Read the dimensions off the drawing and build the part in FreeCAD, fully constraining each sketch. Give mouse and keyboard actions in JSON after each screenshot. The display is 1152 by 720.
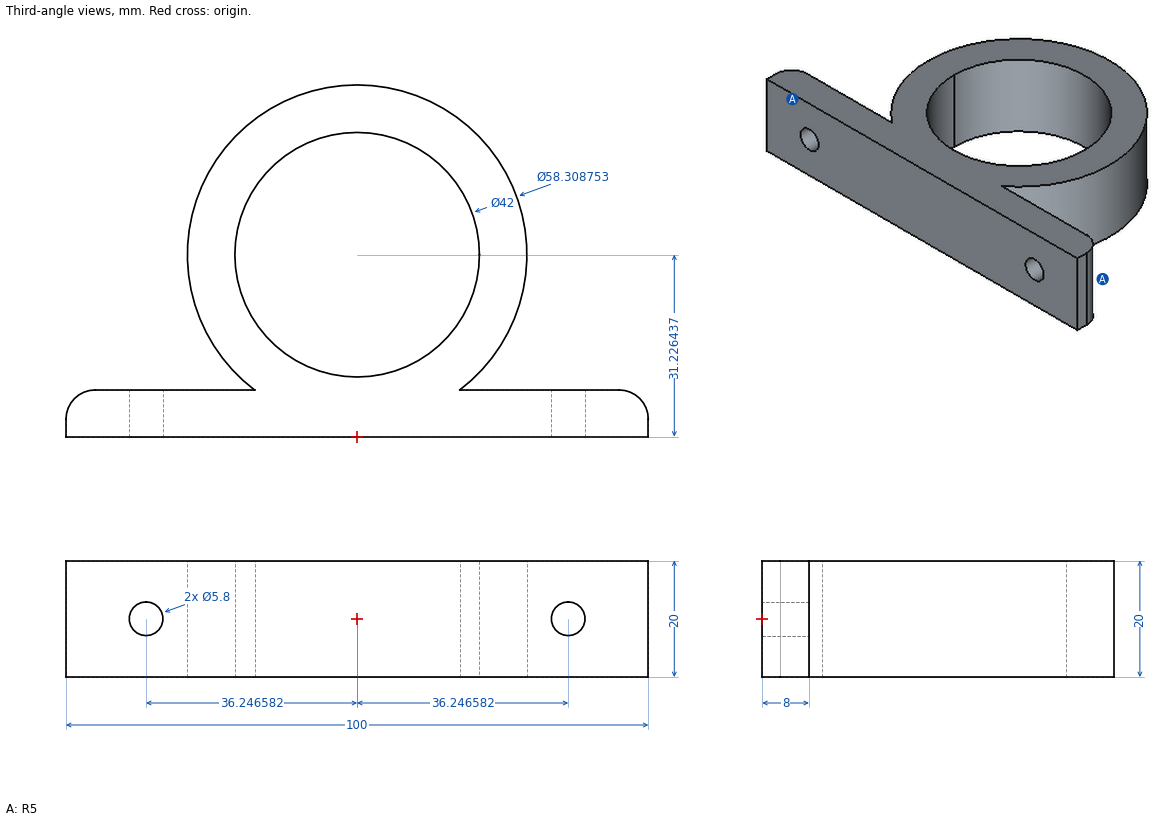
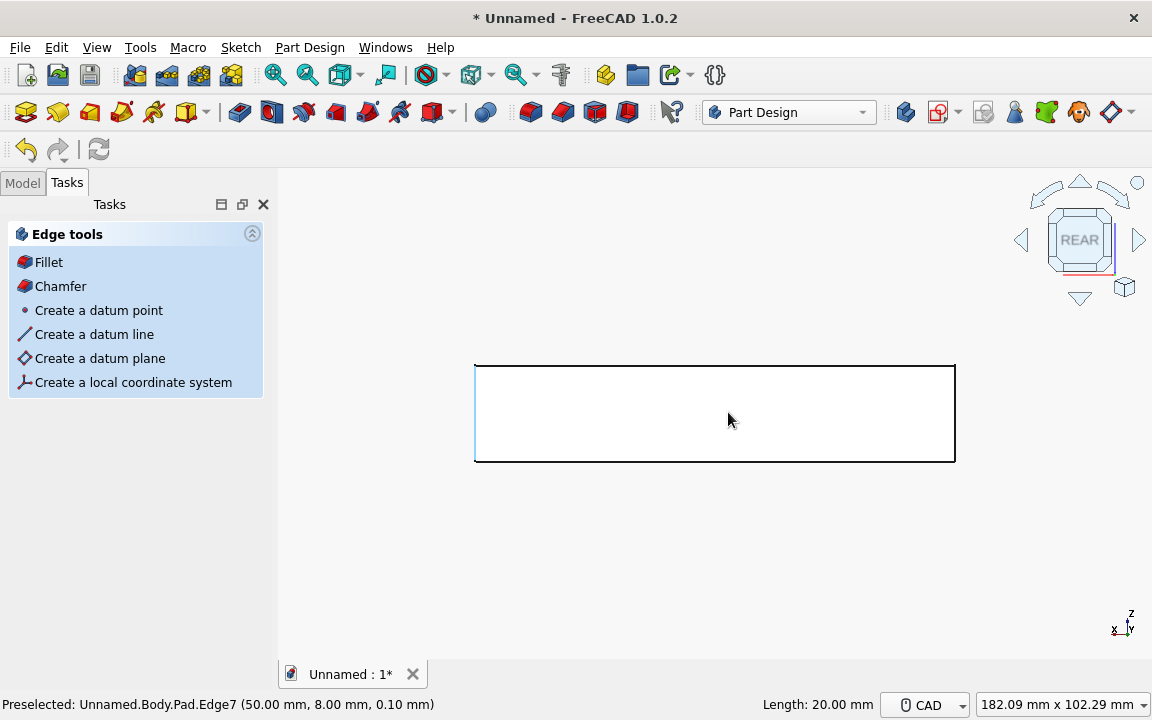
{"action": "left_click", "coordinate": [955, 412], "text": "ctrl"}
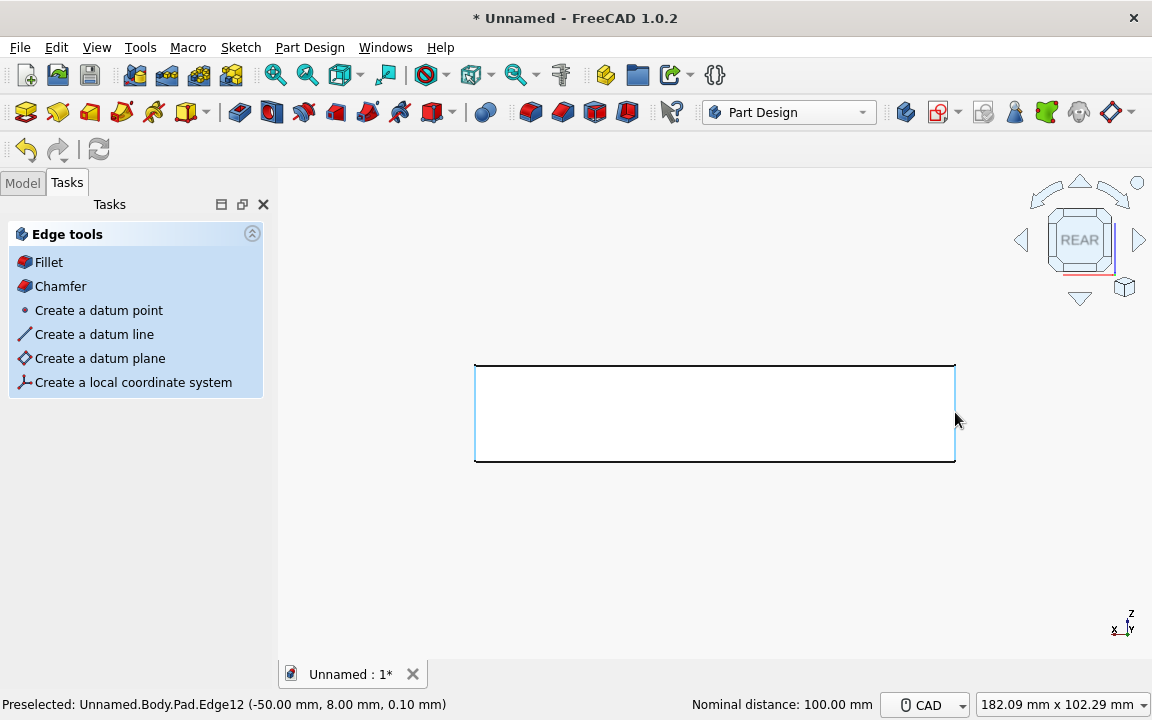
{"action": "left_click", "coordinate": [532, 112]}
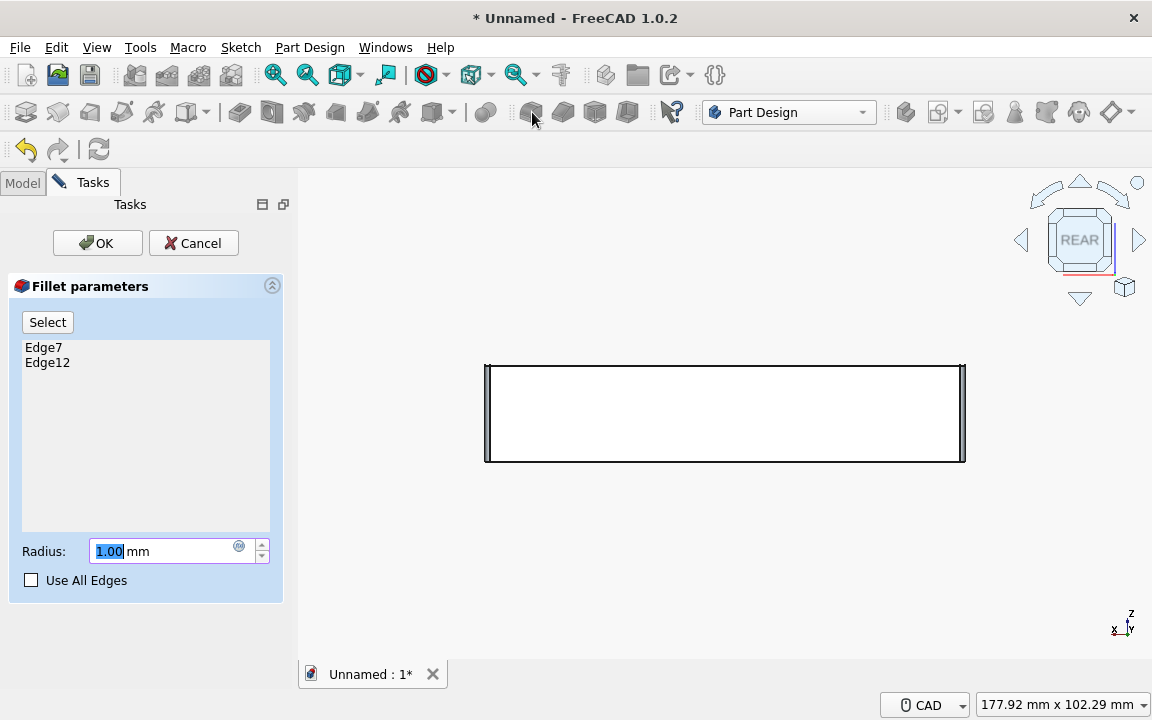
{"action": "type", "text": "5"}
{"action": "key", "text": "Tab"}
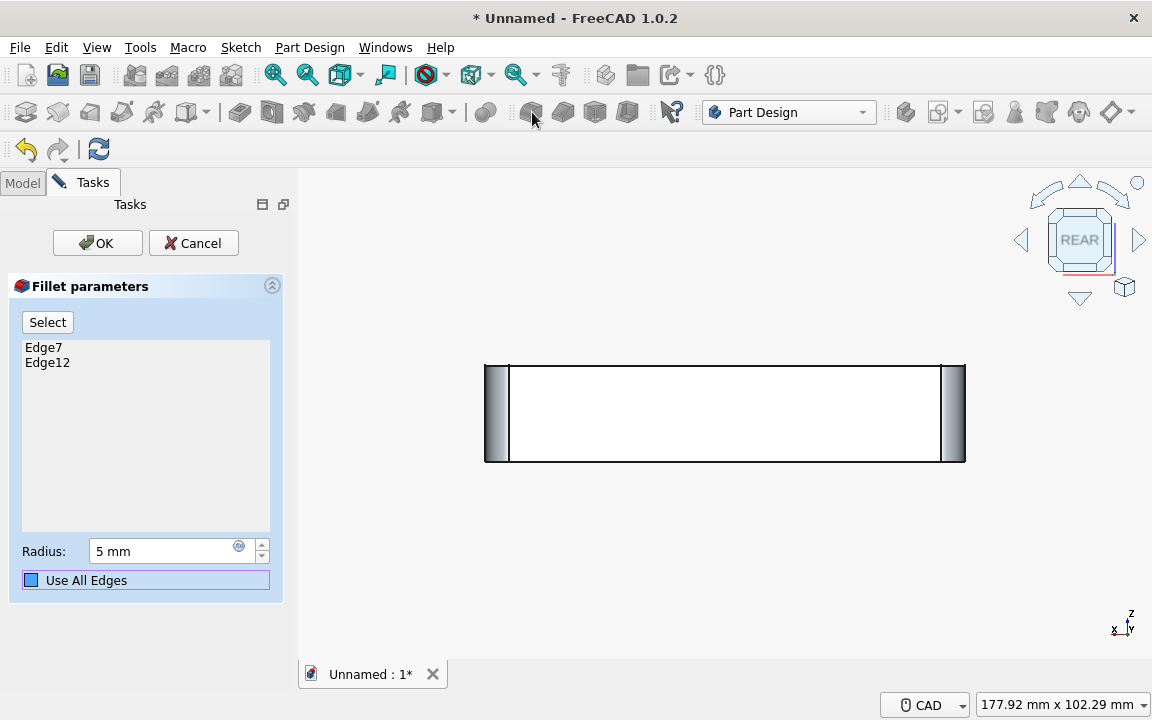
{"action": "left_click", "coordinate": [98, 243]}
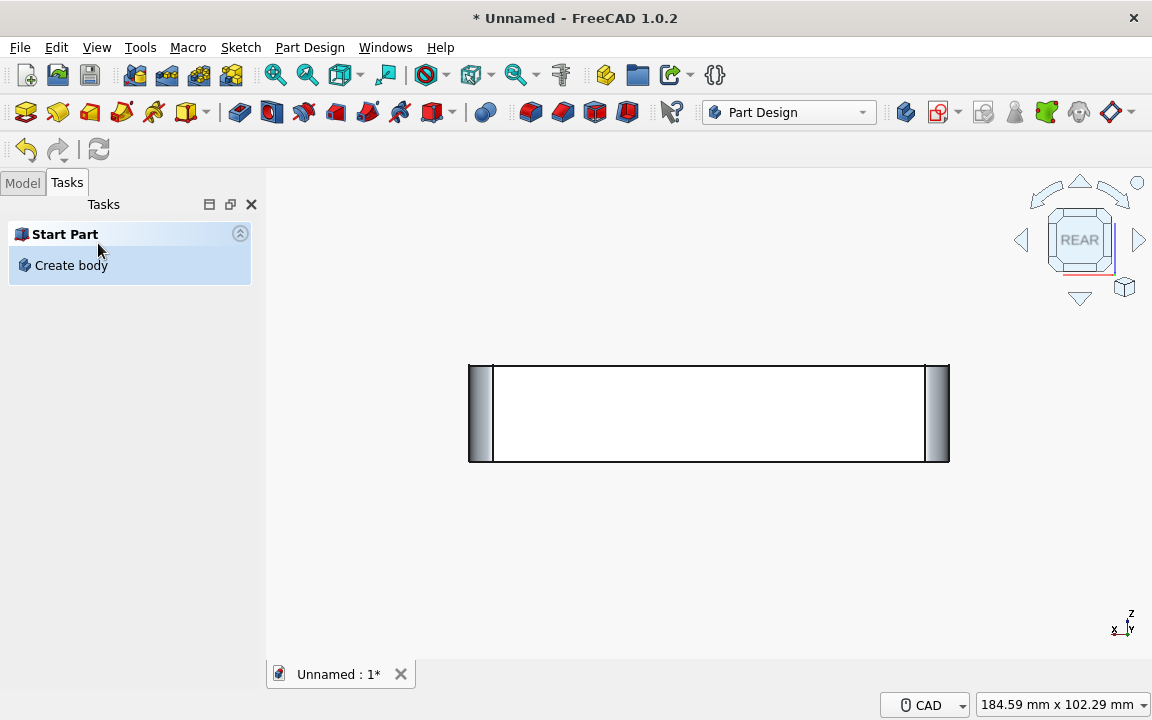
{"action": "key", "text": "0"}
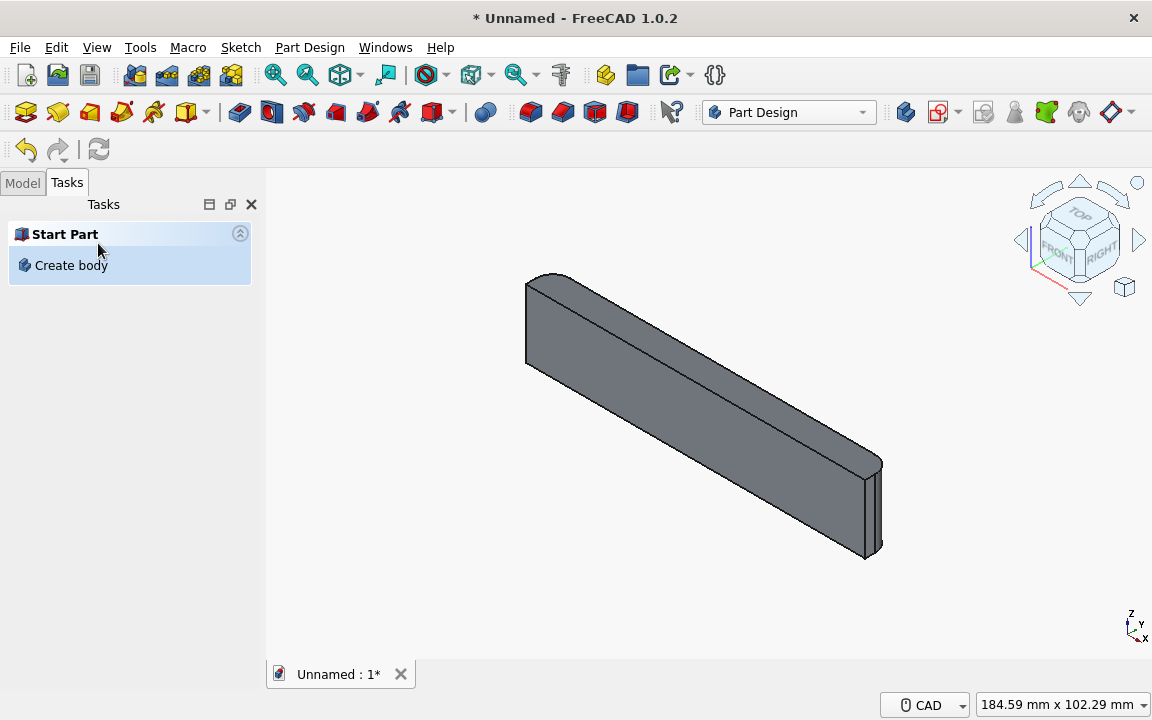
{"action": "left_click", "coordinate": [854, 457]}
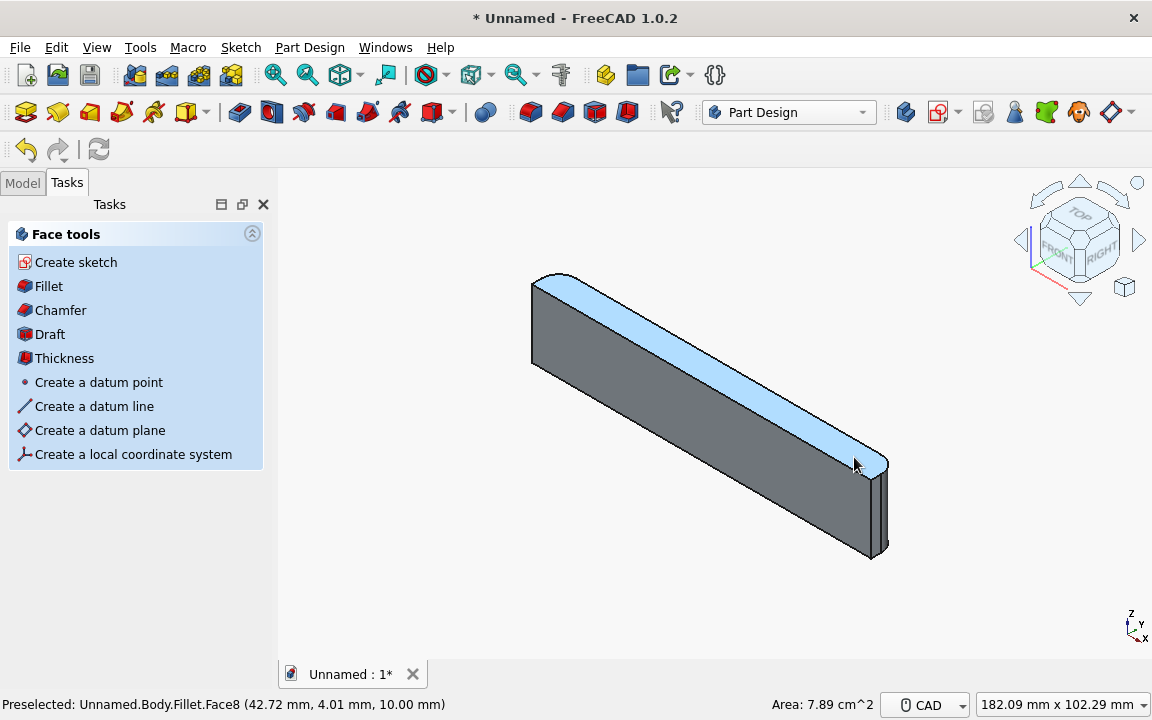
{"action": "left_click", "coordinate": [938, 112]}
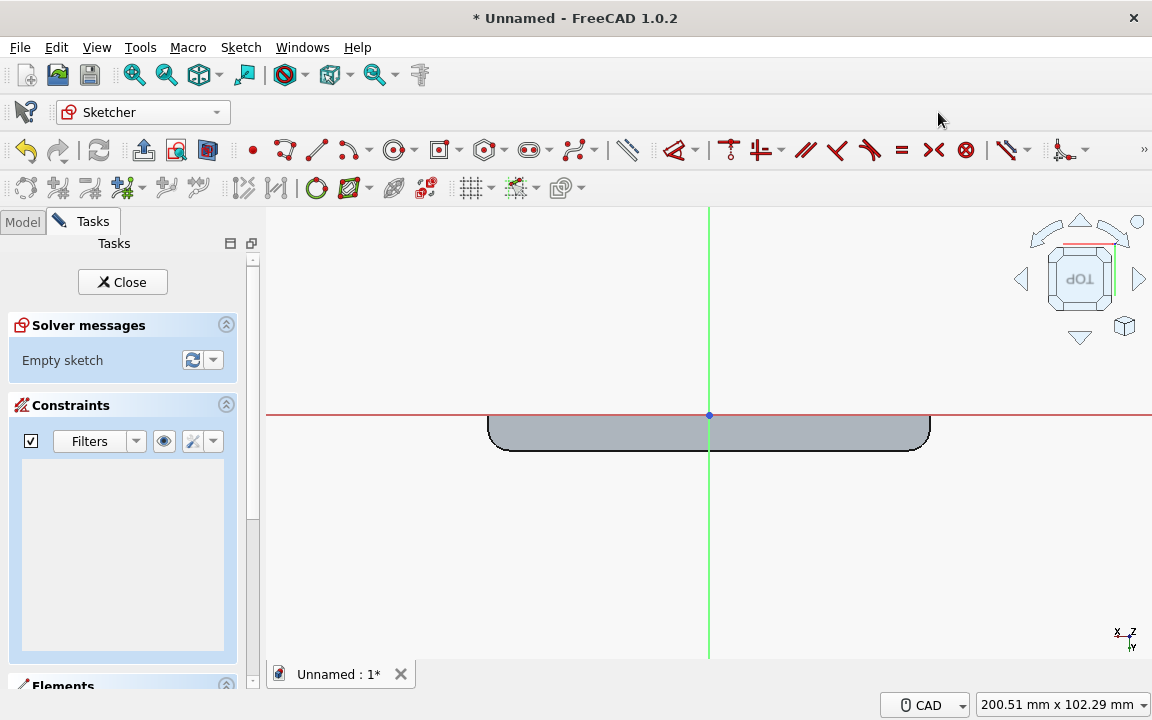
{"action": "scroll", "coordinate": [331, 235], "scroll_direction": "down", "scroll_amount": 1}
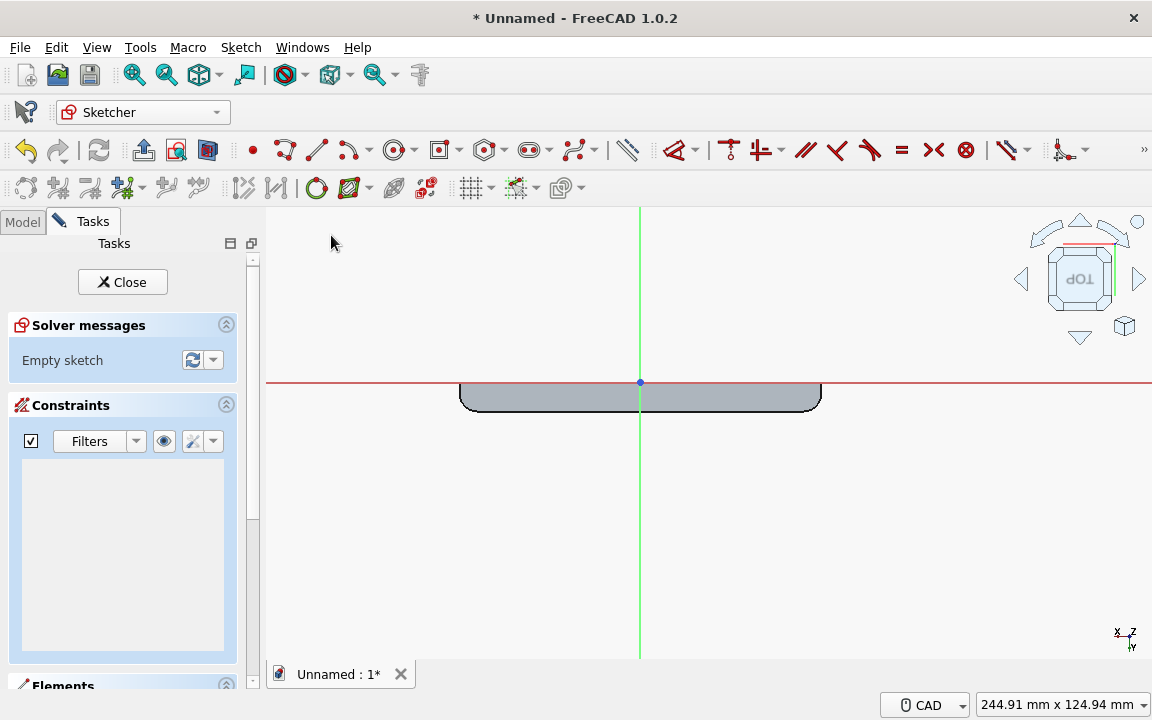
{"action": "left_click", "coordinate": [394, 150]}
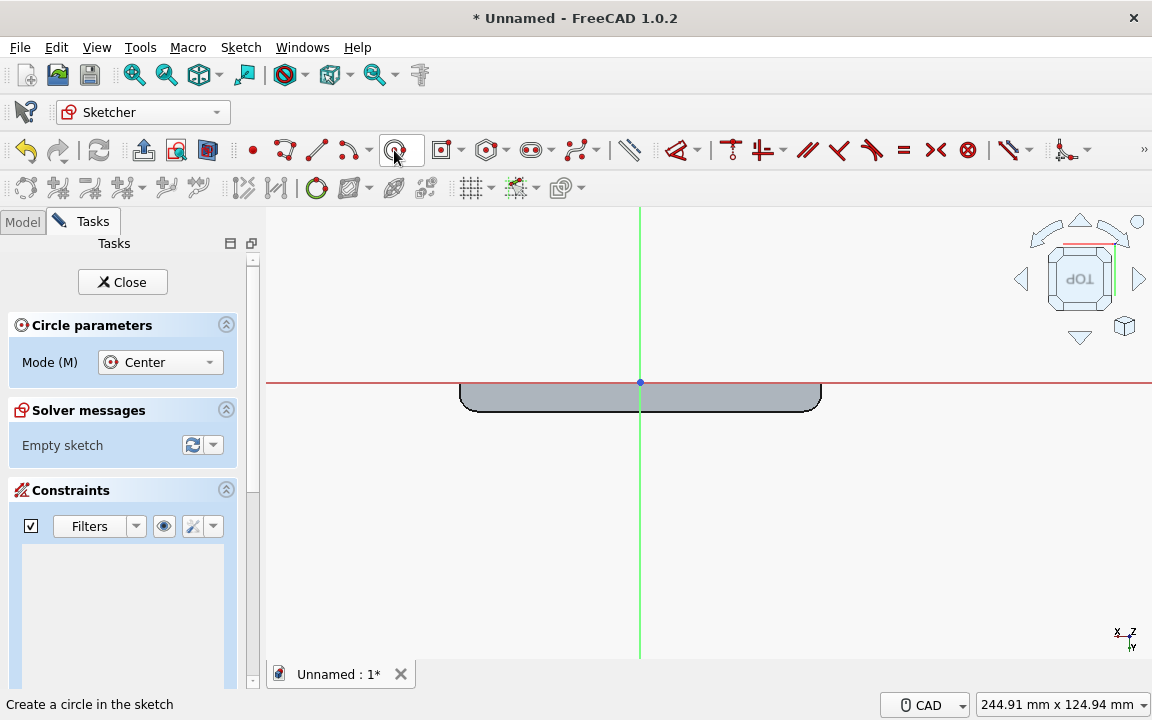
{"action": "left_click", "coordinate": [640, 496]}
{"action": "left_click", "coordinate": [715, 421]}
{"action": "key", "text": "Escape"}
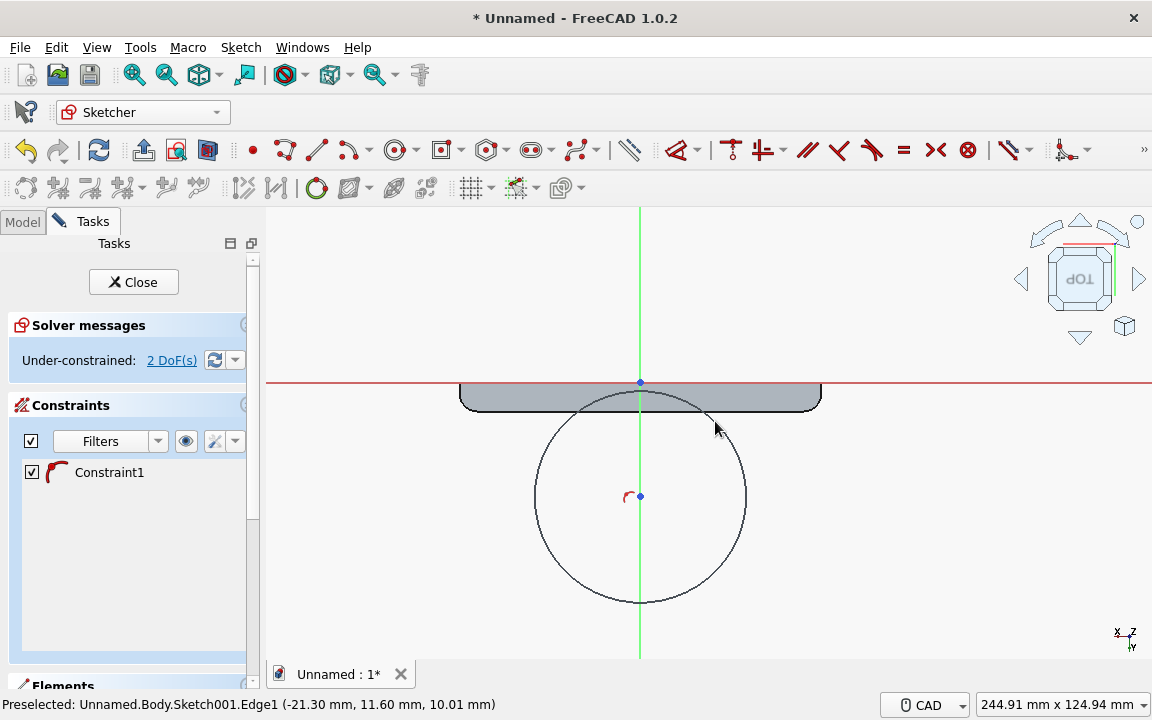
{"action": "left_click", "coordinate": [676, 150]}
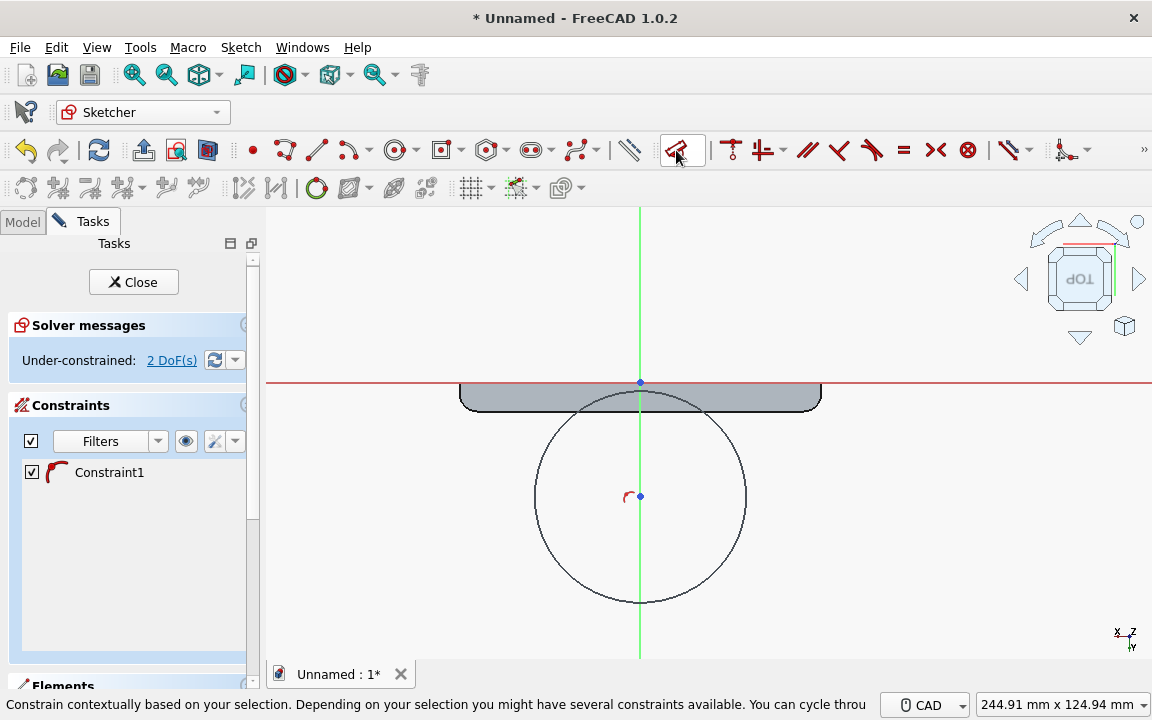
{"action": "left_click", "coordinate": [715, 422]}
{"action": "left_click", "coordinate": [738, 399]}